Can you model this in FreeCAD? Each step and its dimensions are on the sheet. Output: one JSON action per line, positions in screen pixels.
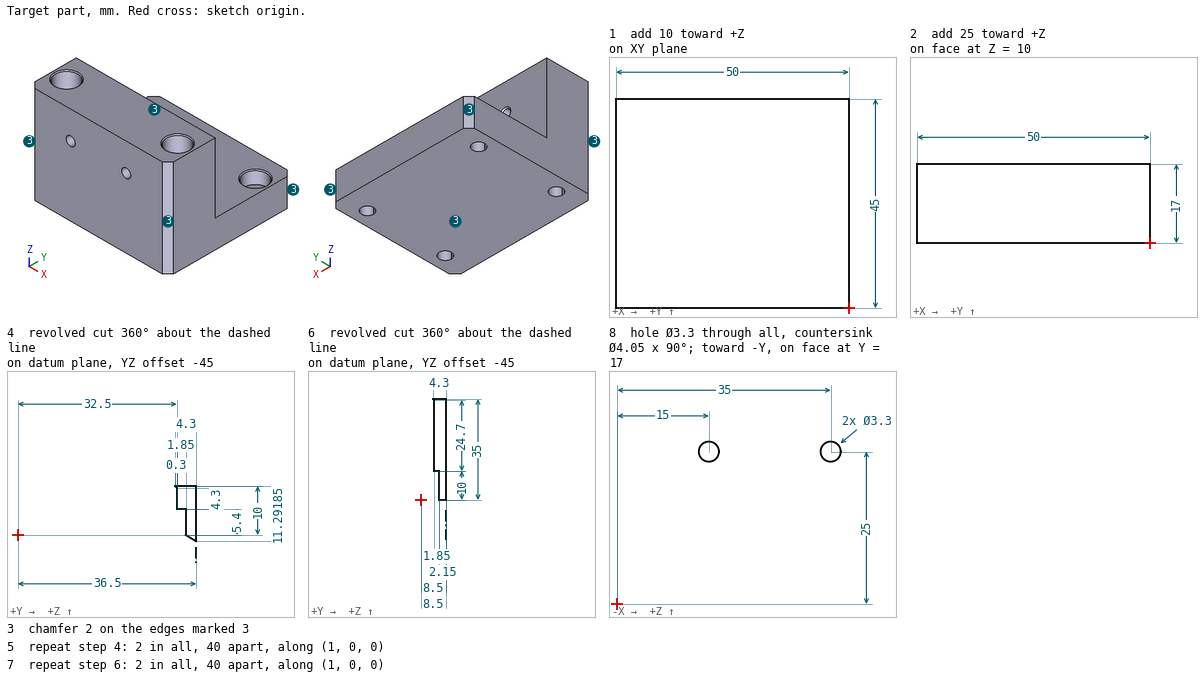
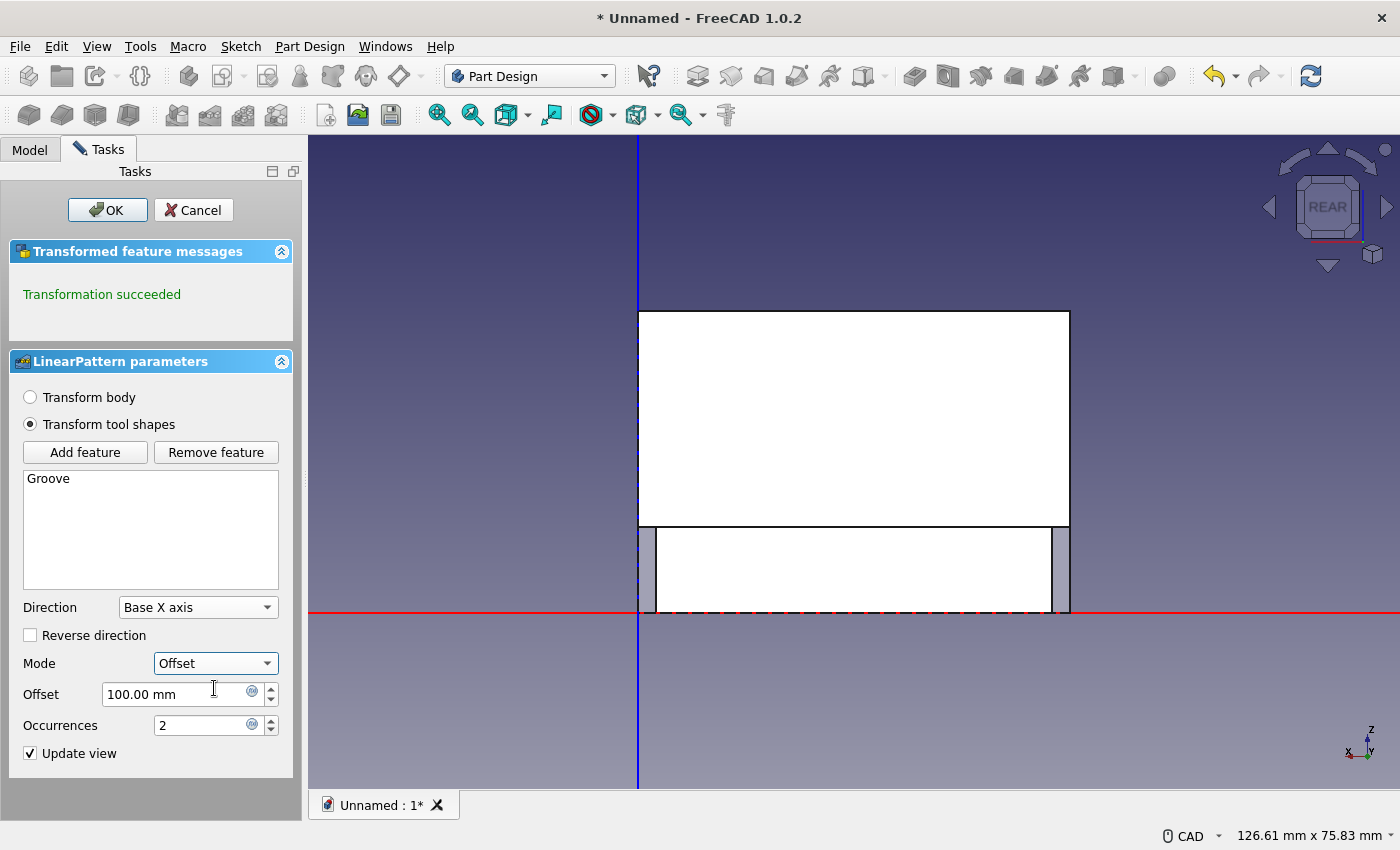
{"action": "triple_click", "coordinate": [184, 694]}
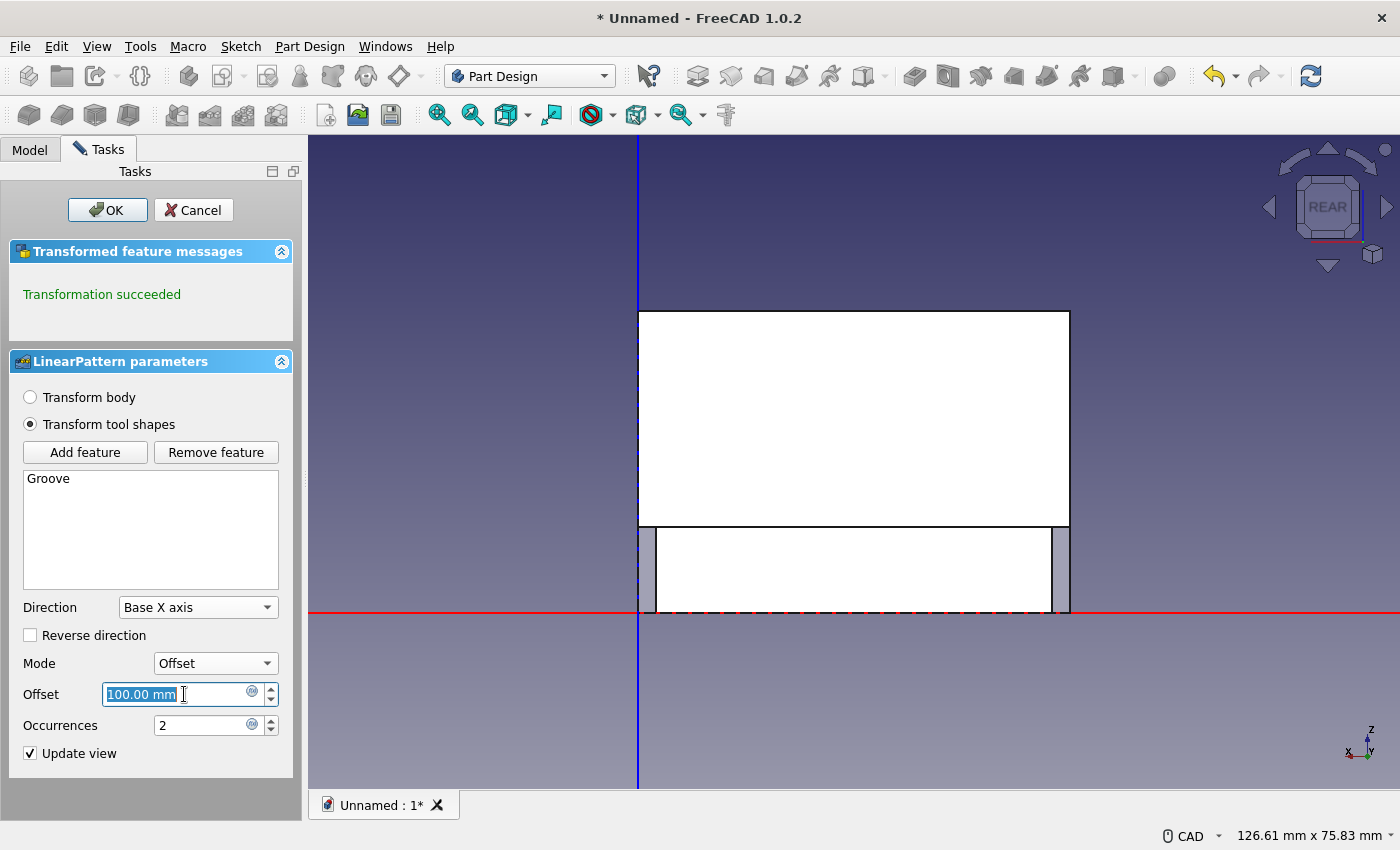
{"action": "type", "text": "40"}
{"action": "key", "text": "Tab"}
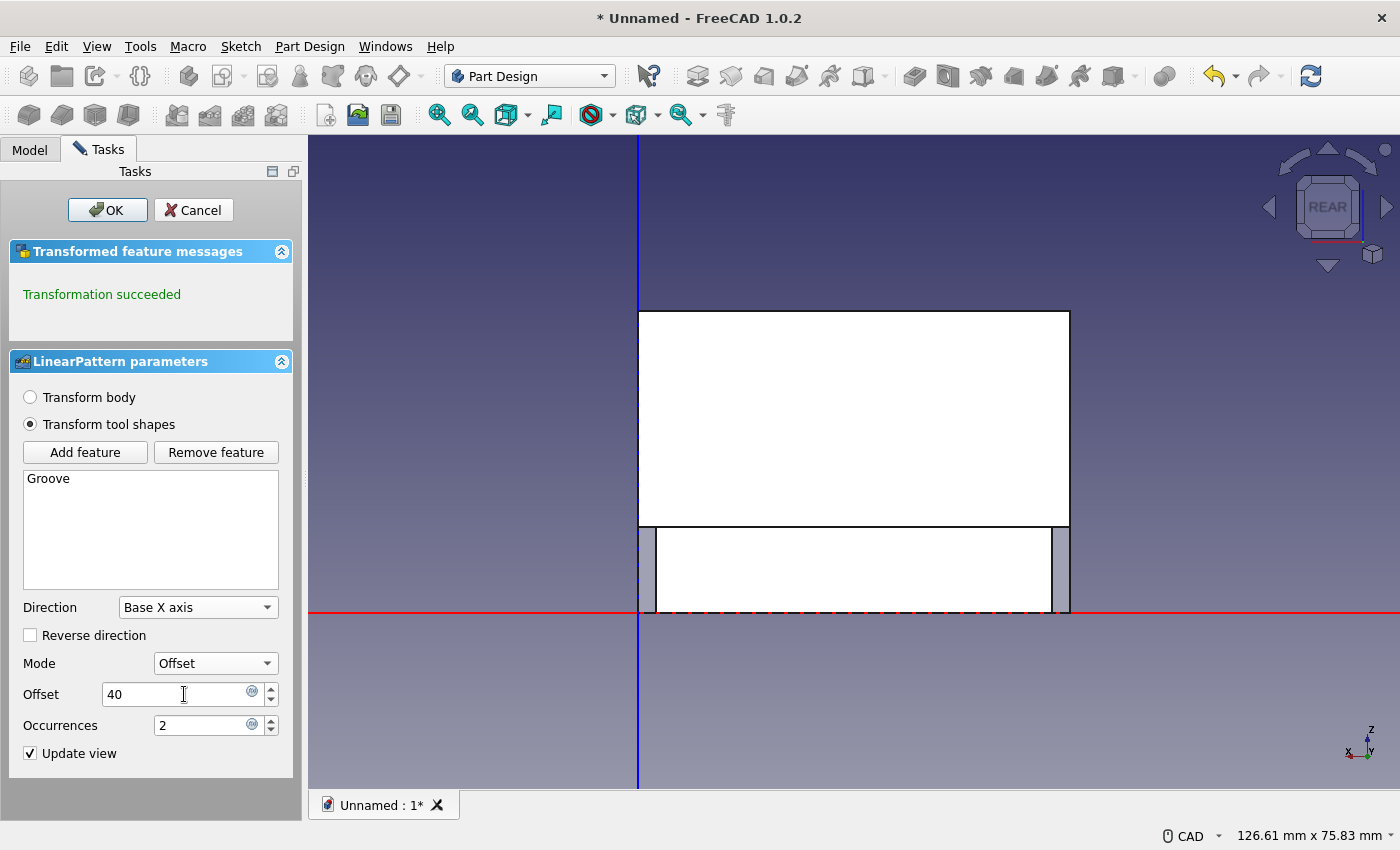
{"action": "triple_click", "coordinate": [210, 726]}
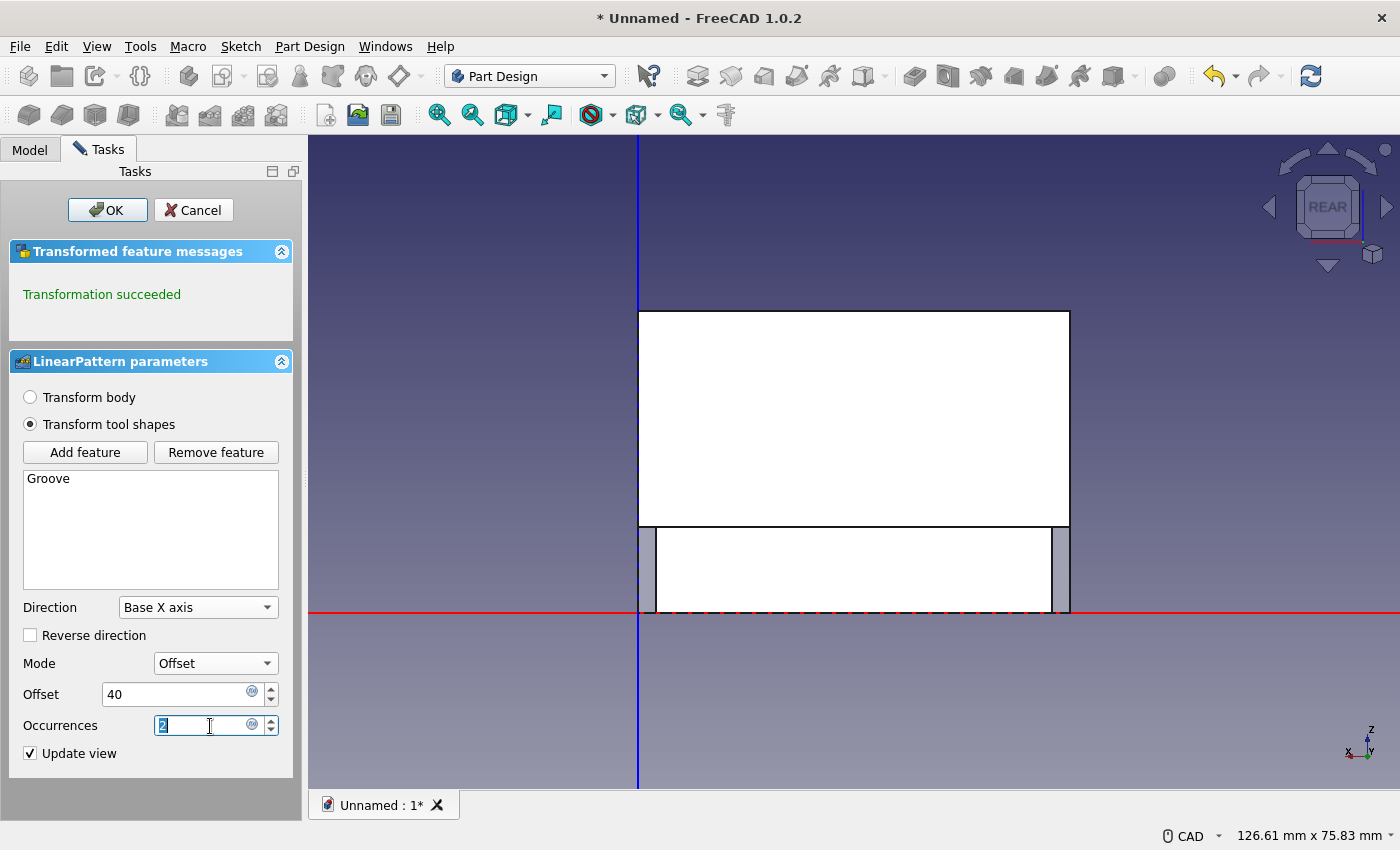
{"action": "type", "text": "2"}
{"action": "key", "text": "Tab"}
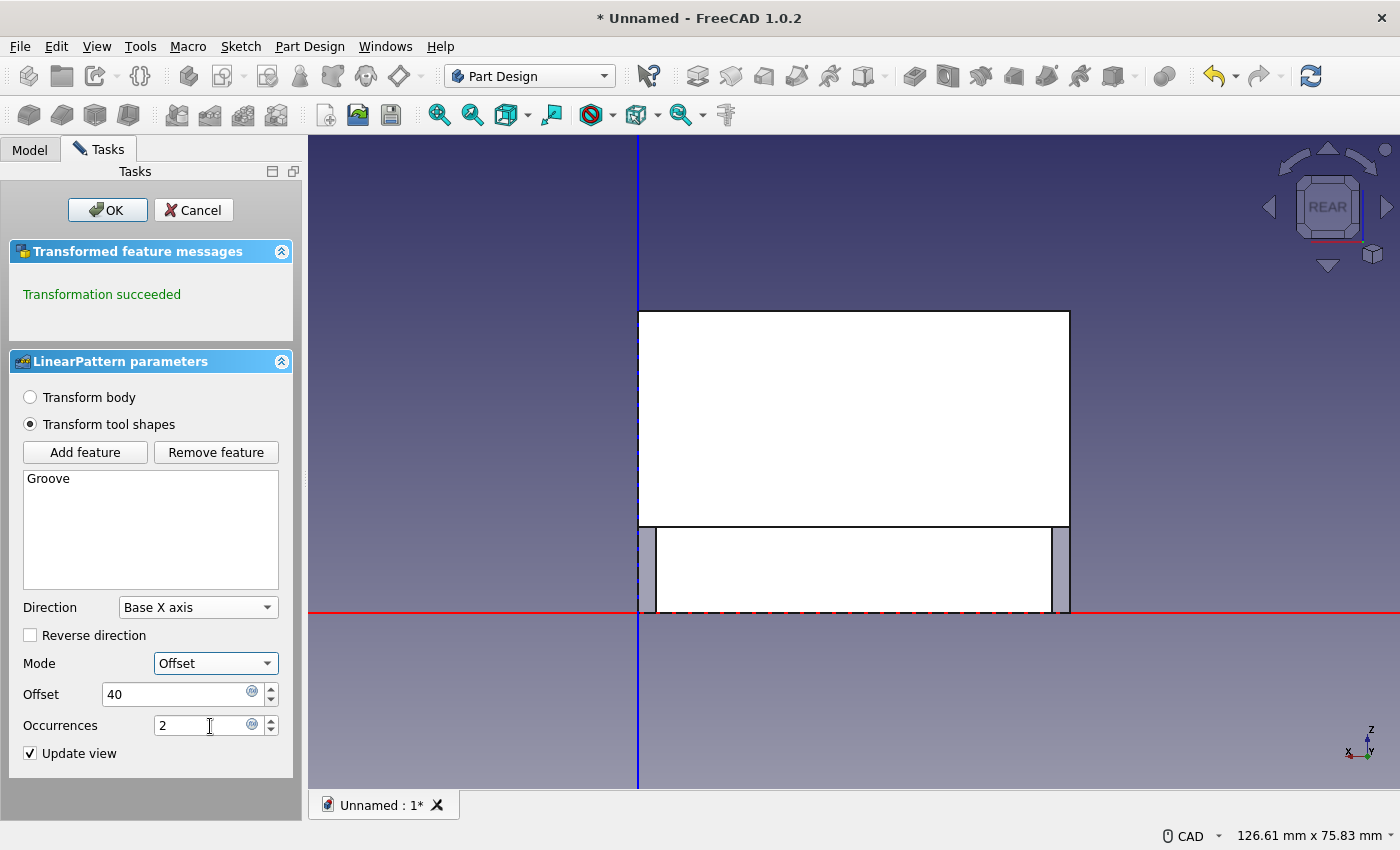
{"action": "left_click", "coordinate": [108, 210]}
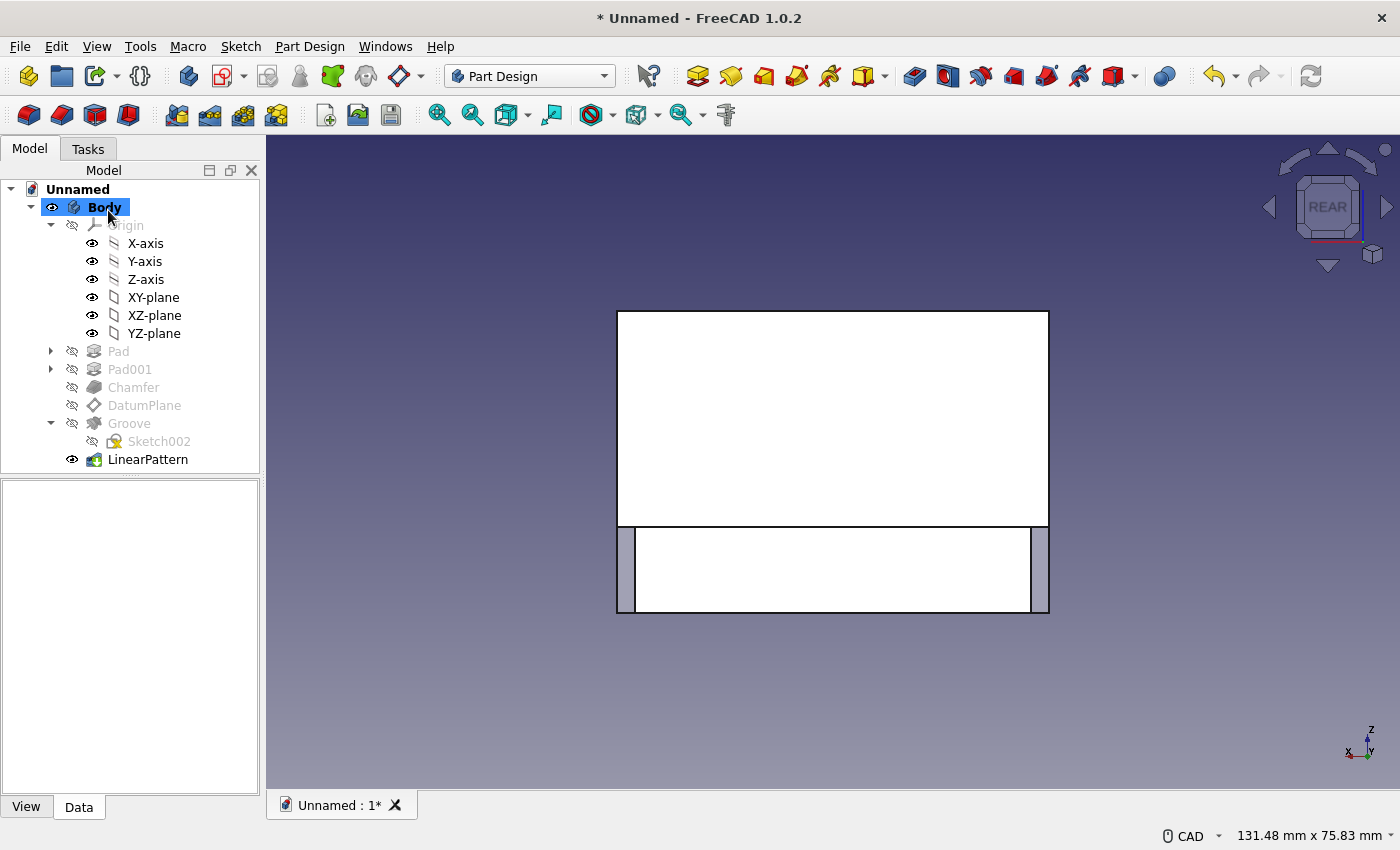
{"action": "left_click", "coordinate": [137, 333]}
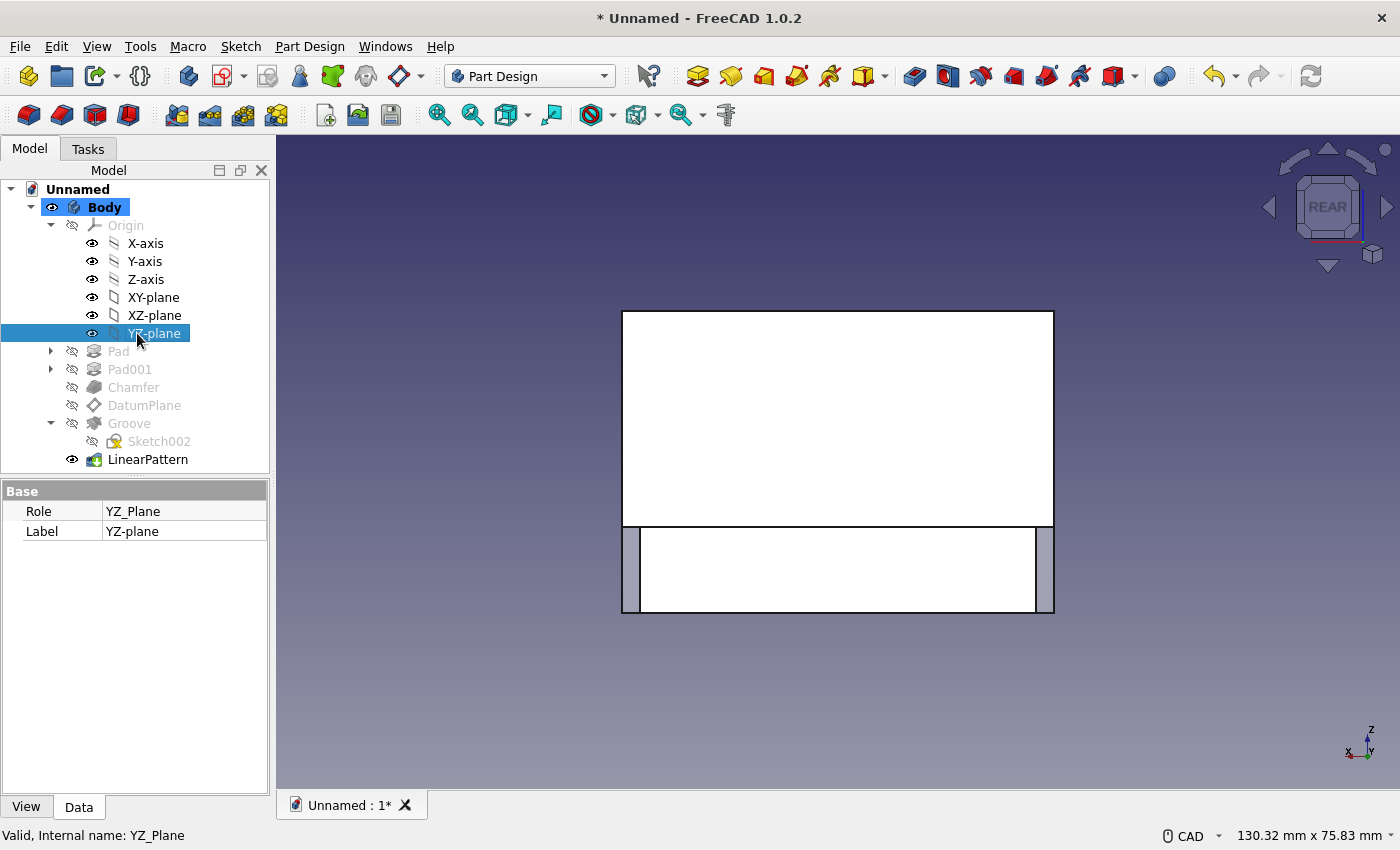
{"action": "left_click", "coordinate": [398, 76]}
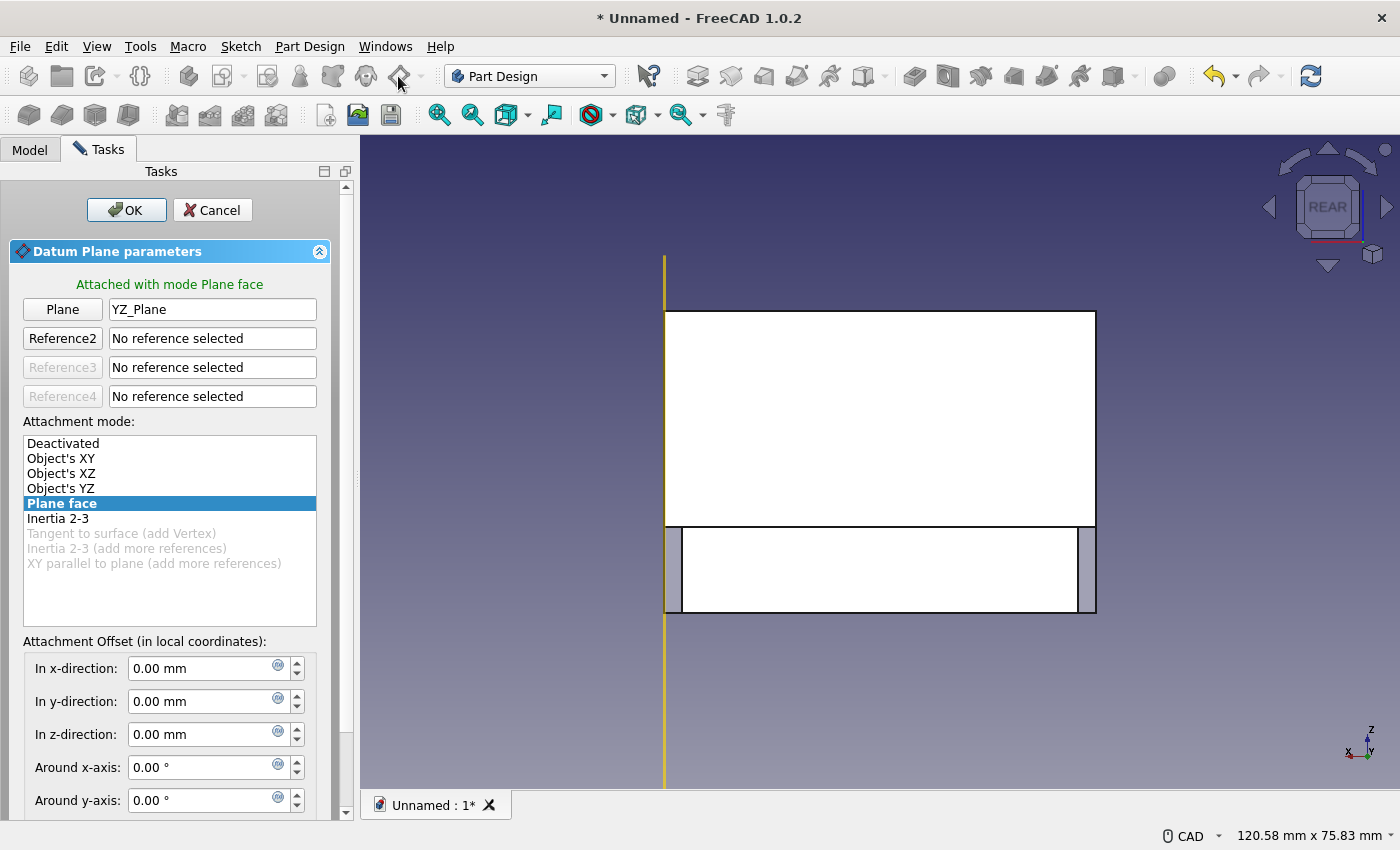
{"action": "triple_click", "coordinate": [210, 734]}